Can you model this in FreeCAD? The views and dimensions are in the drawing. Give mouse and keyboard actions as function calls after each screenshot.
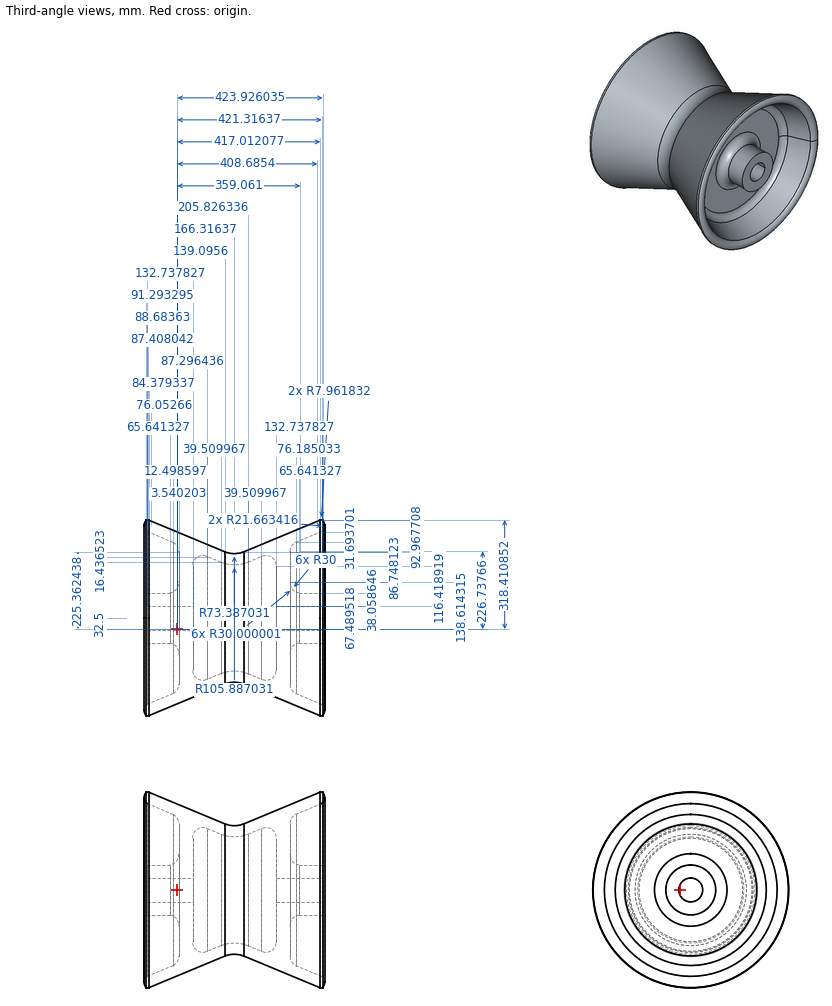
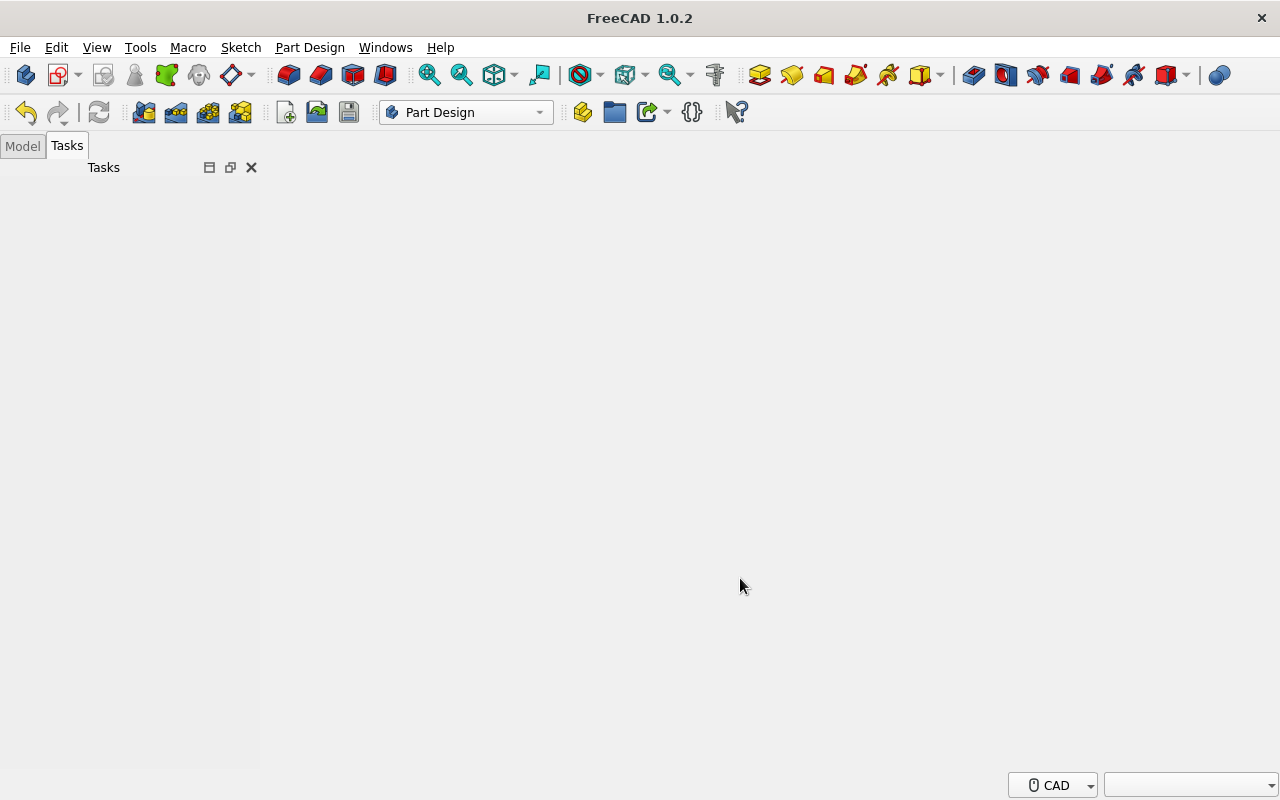
key(ctrl+n)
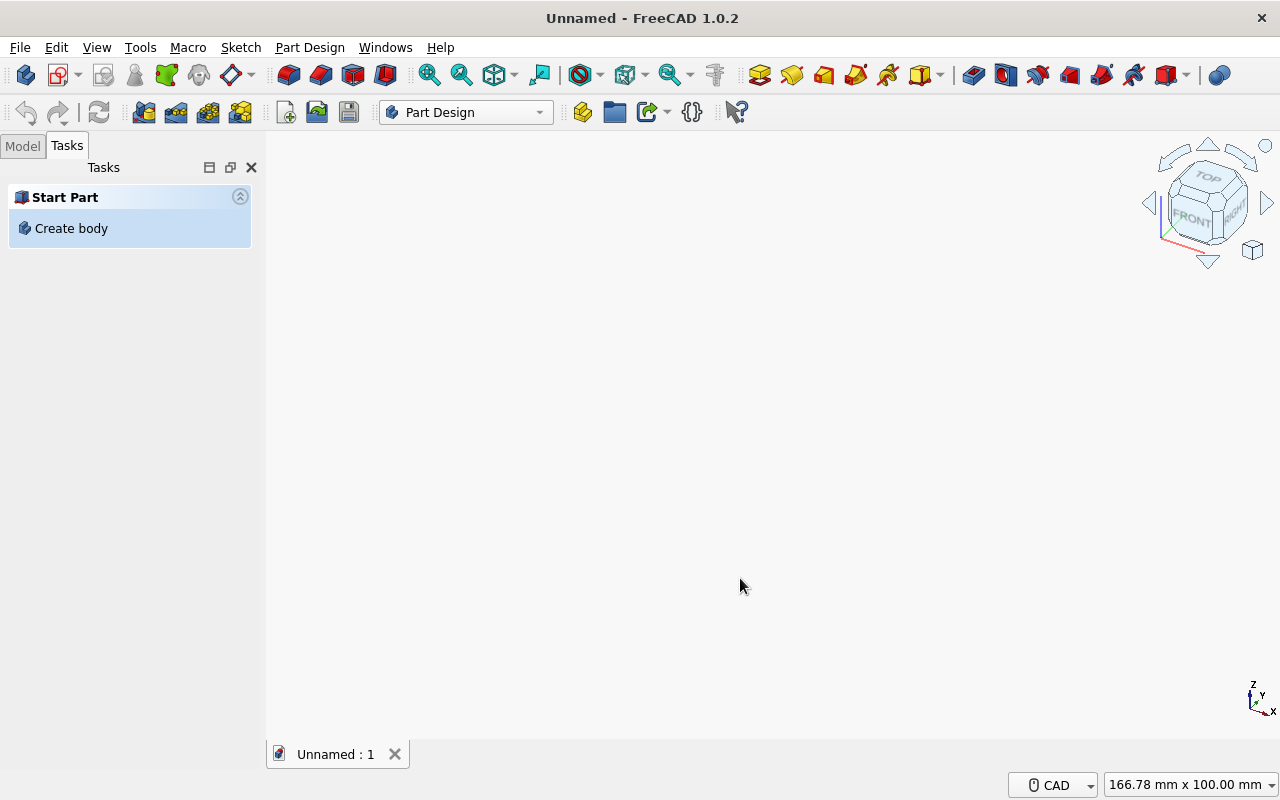
click(58, 76)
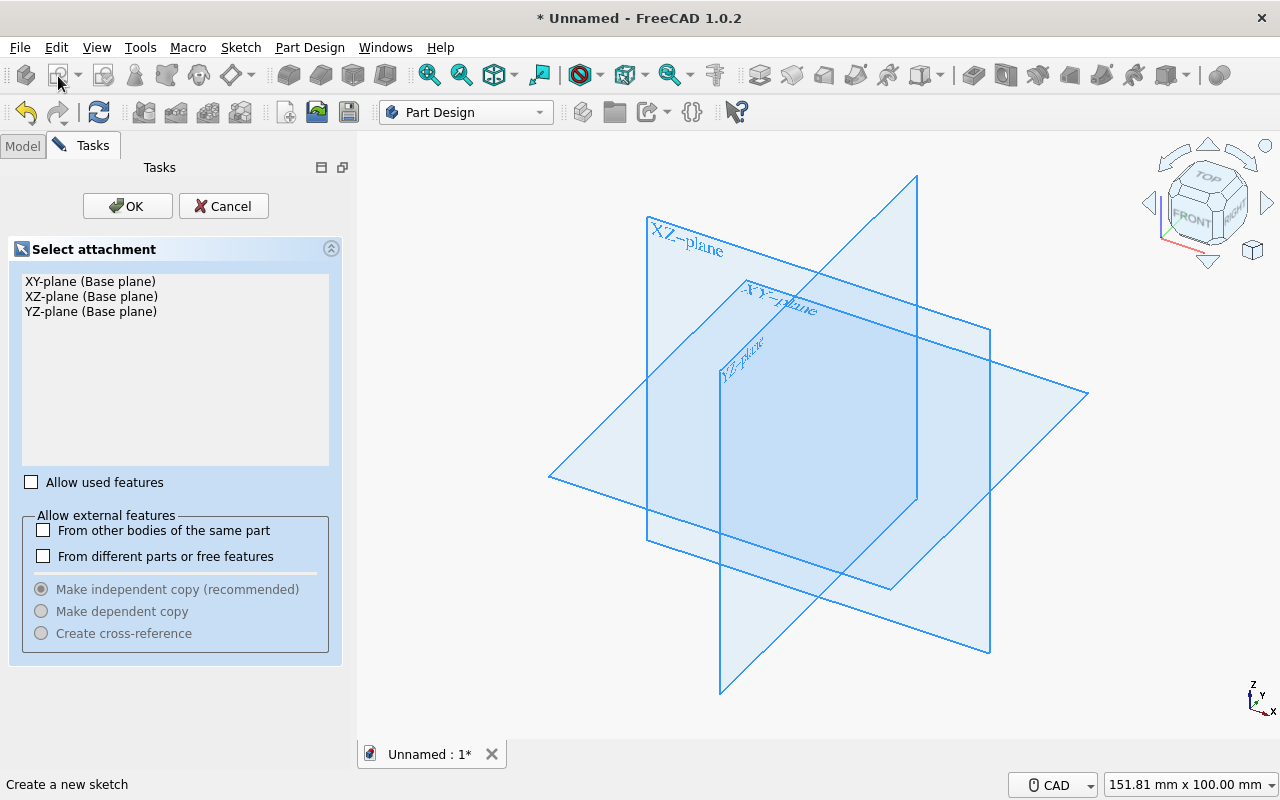
click(82, 282)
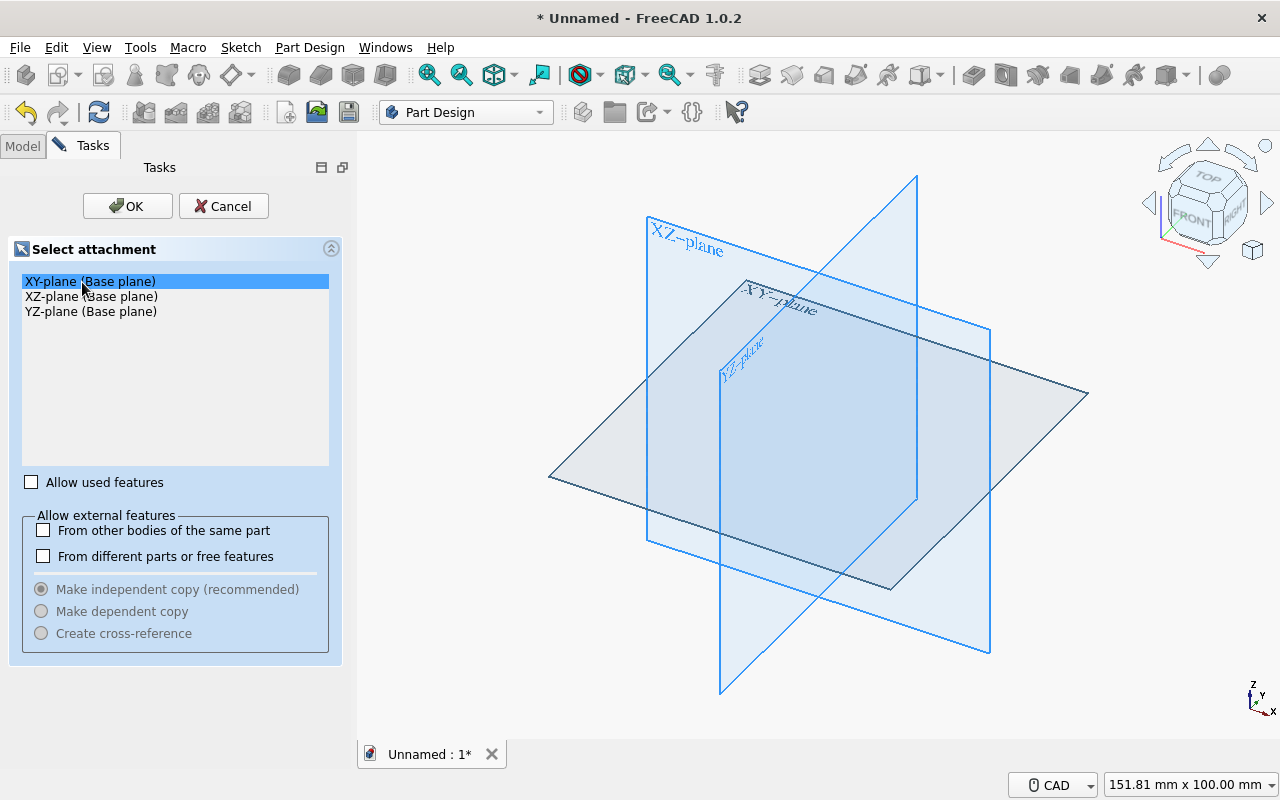
click(128, 206)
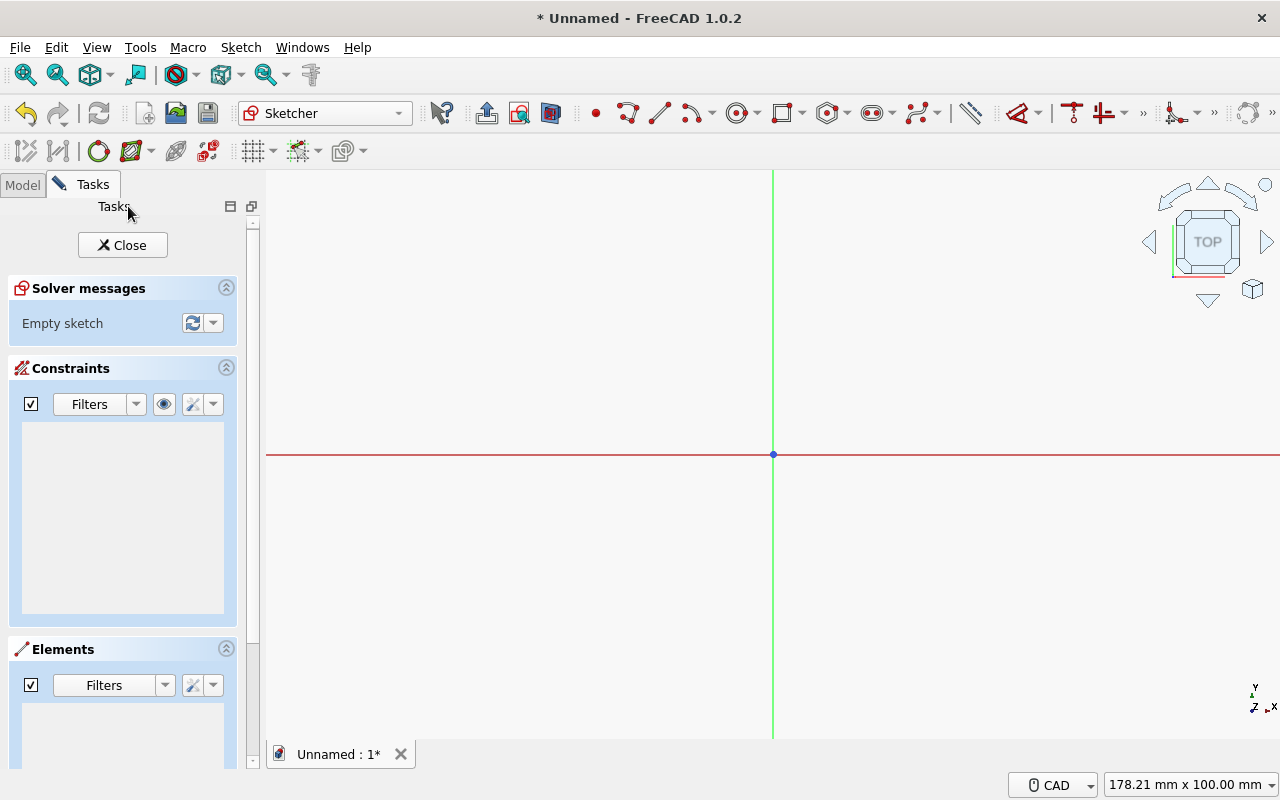
scroll(504, 634, down, 9)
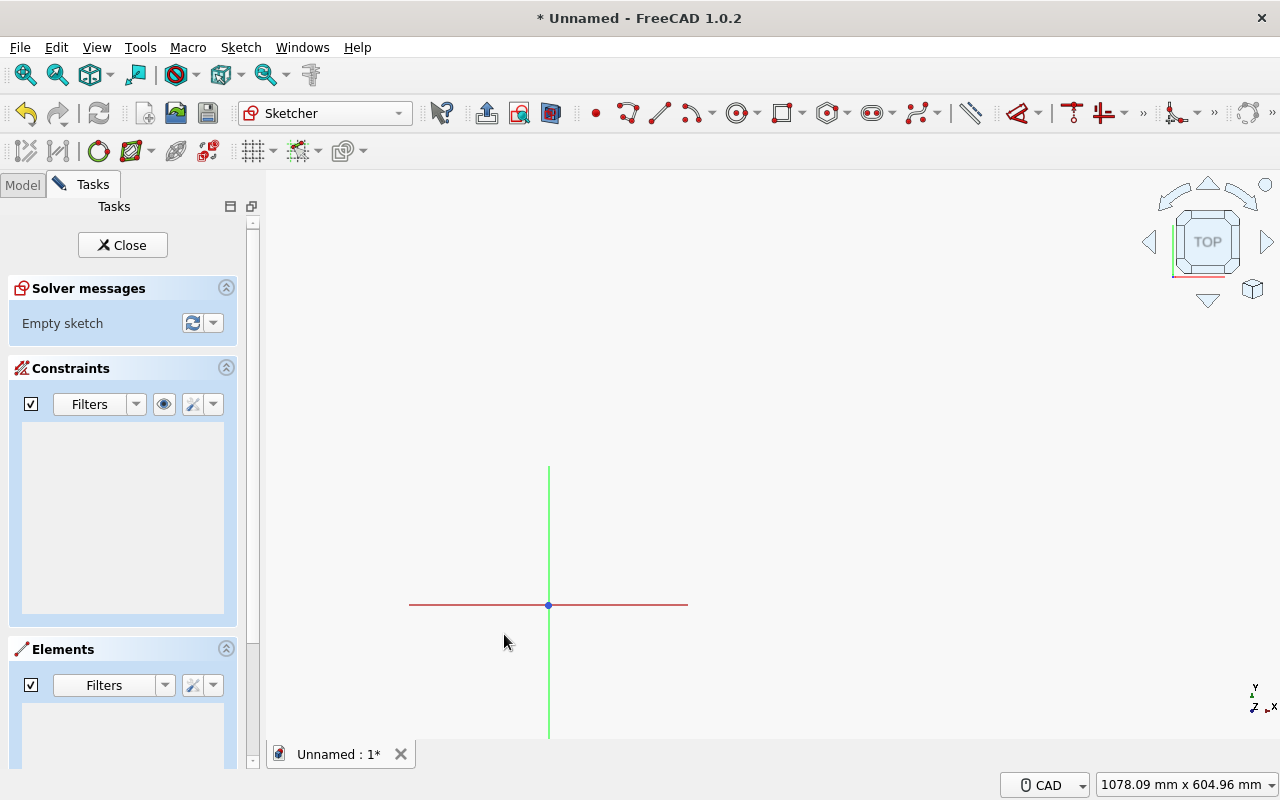
click(628, 114)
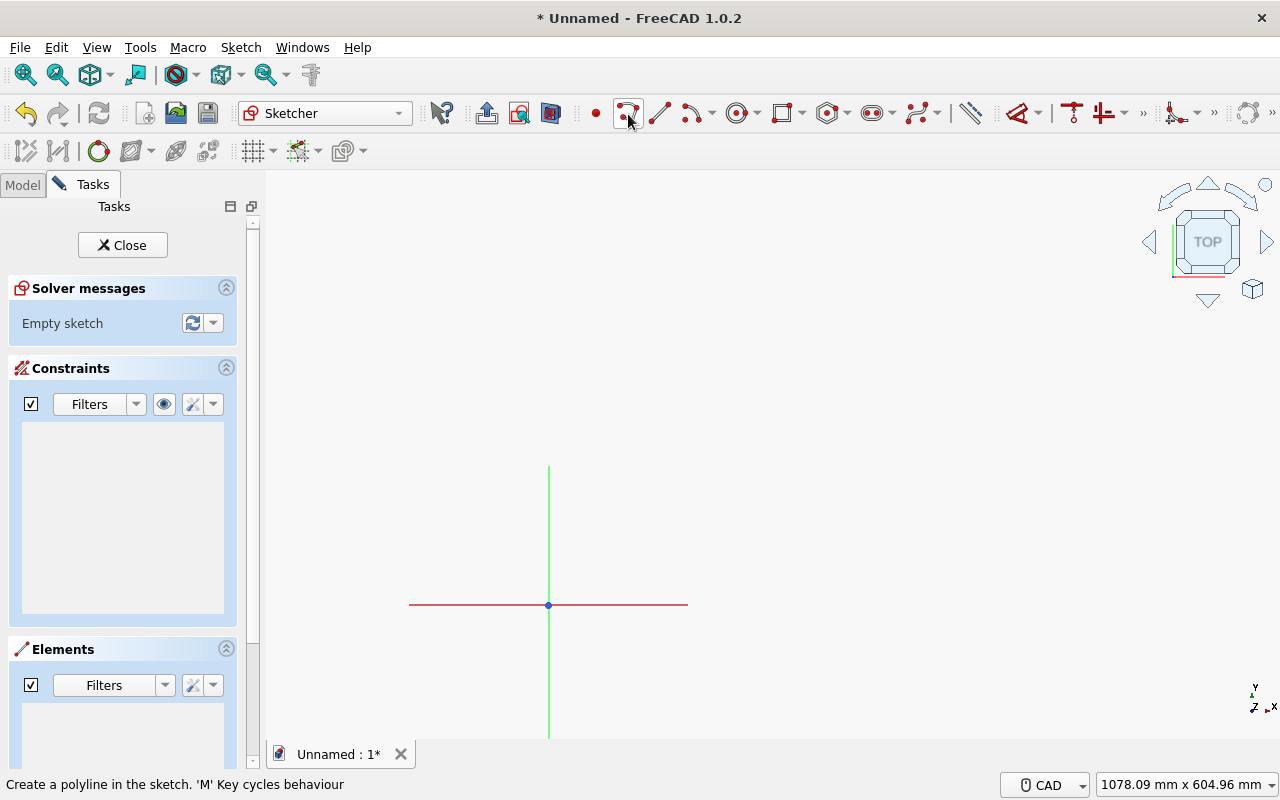
click(820, 432)
click(820, 542)
click(945, 542)
click(945, 506)
click(883, 506)
right_click(883, 506)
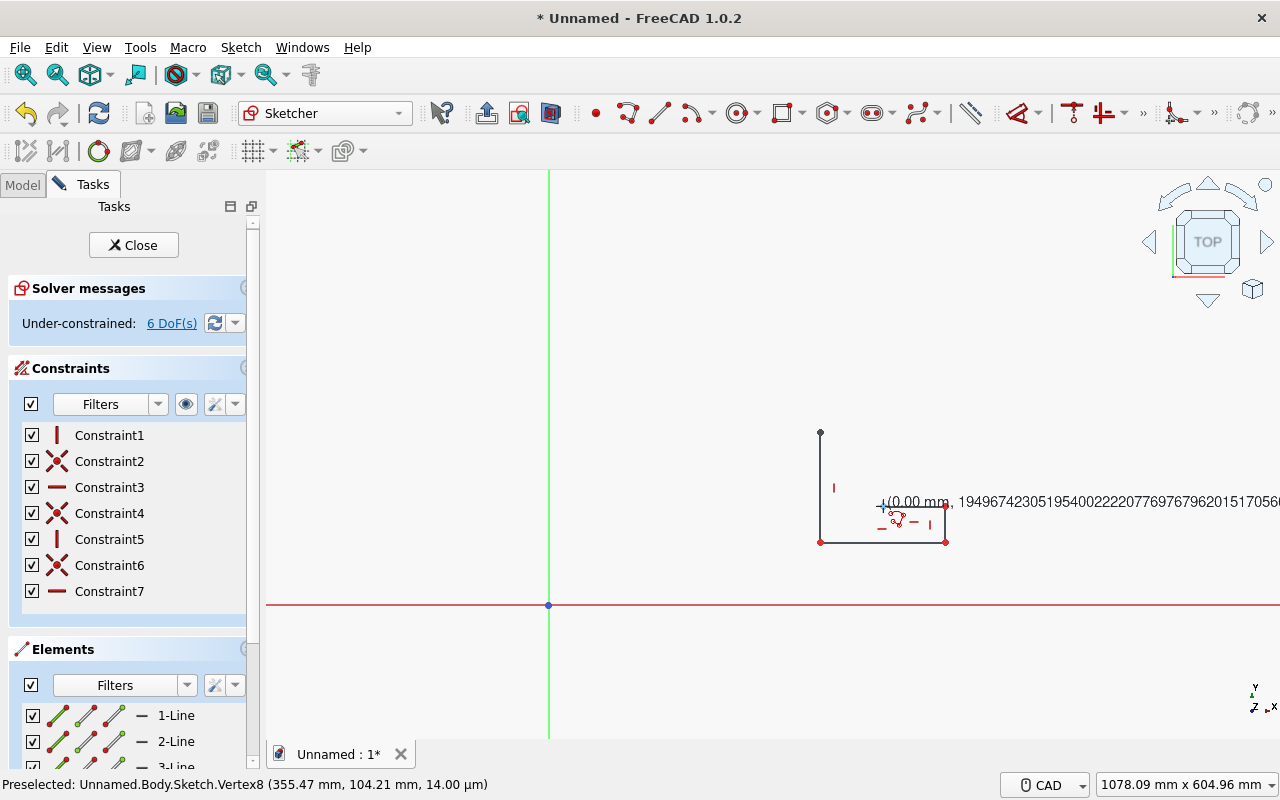
click(660, 114)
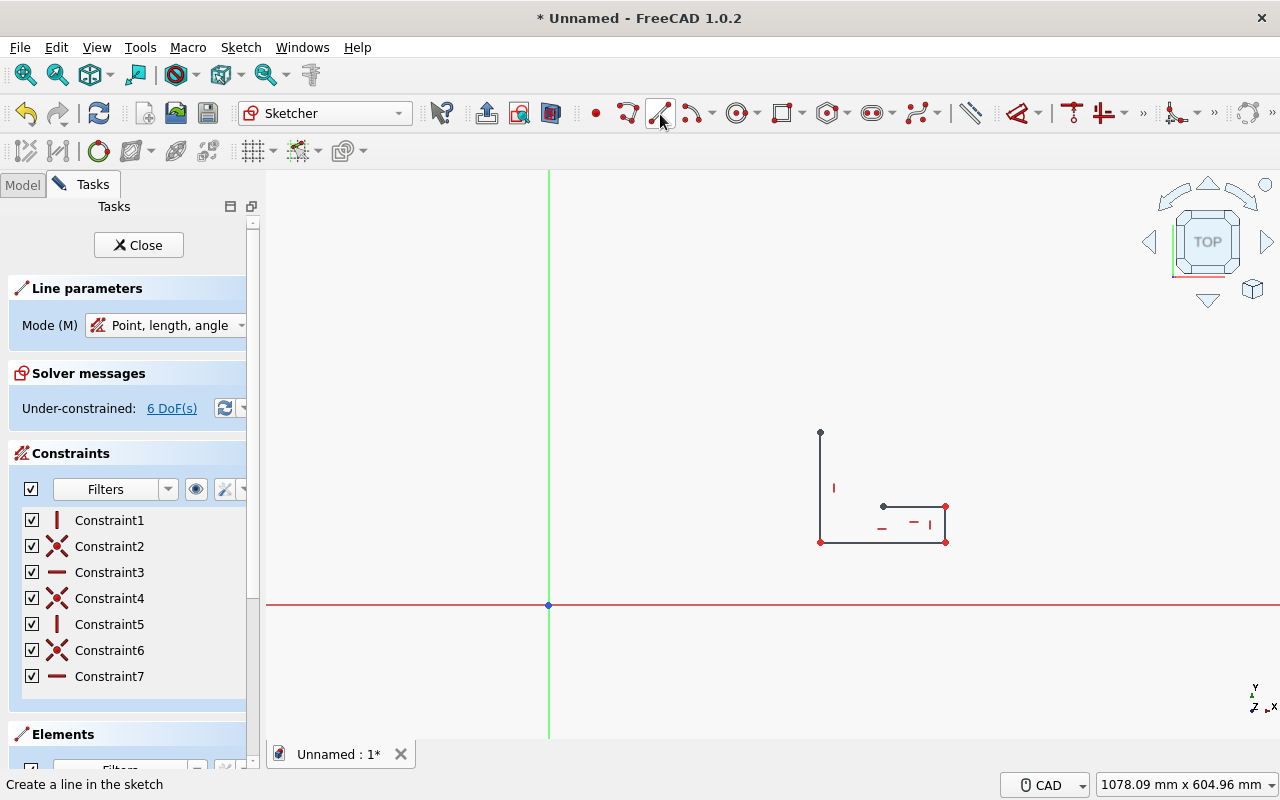
click(858, 475)
click(858, 393)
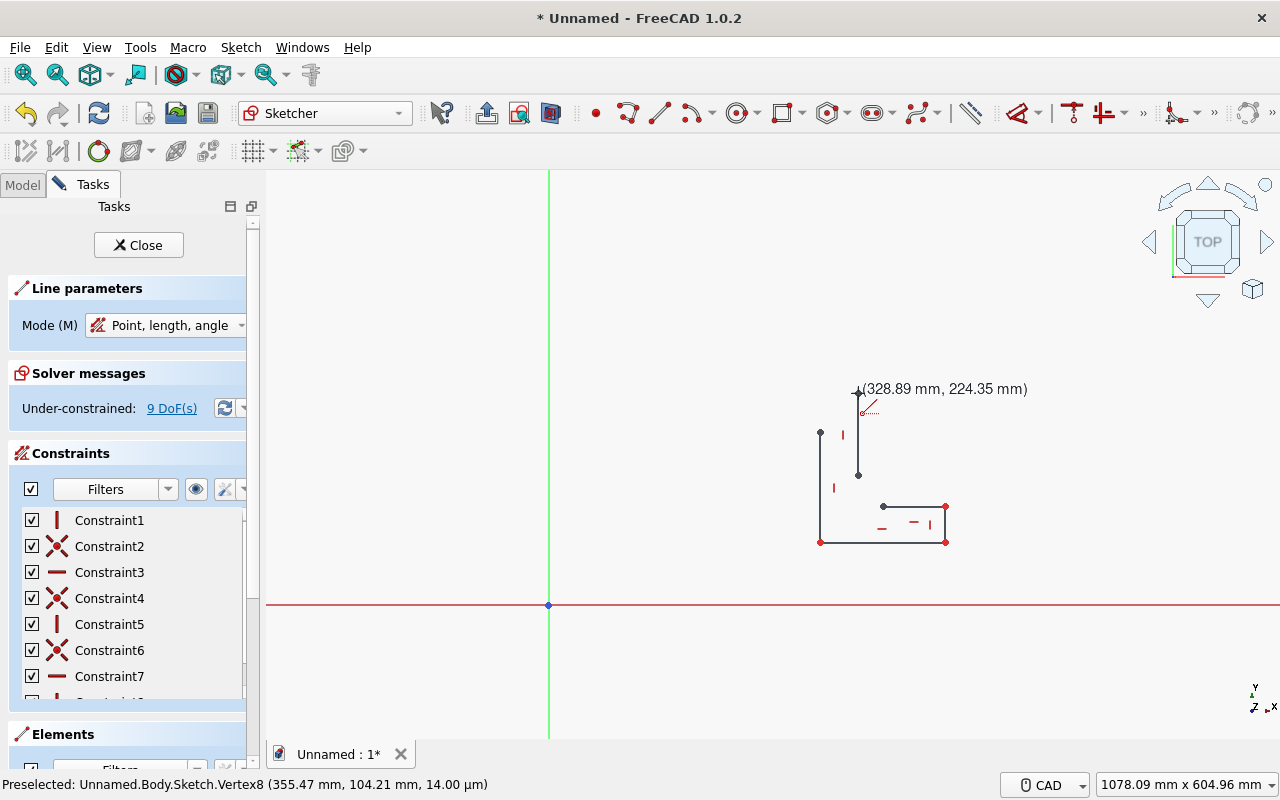
click(873, 367)
click(945, 337)